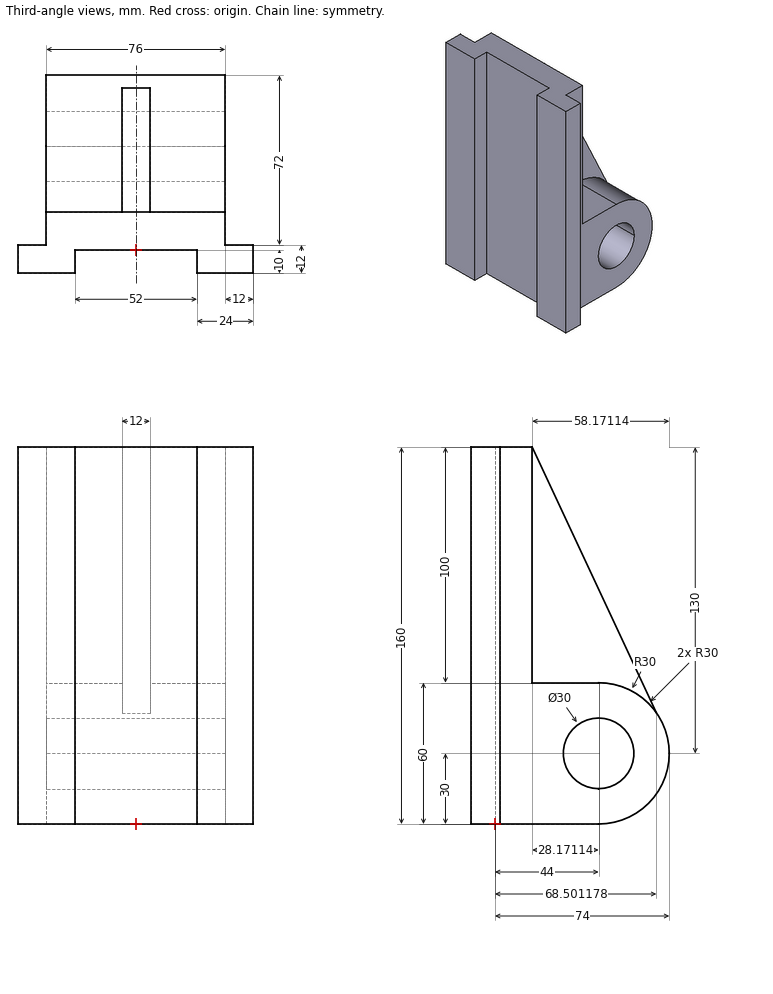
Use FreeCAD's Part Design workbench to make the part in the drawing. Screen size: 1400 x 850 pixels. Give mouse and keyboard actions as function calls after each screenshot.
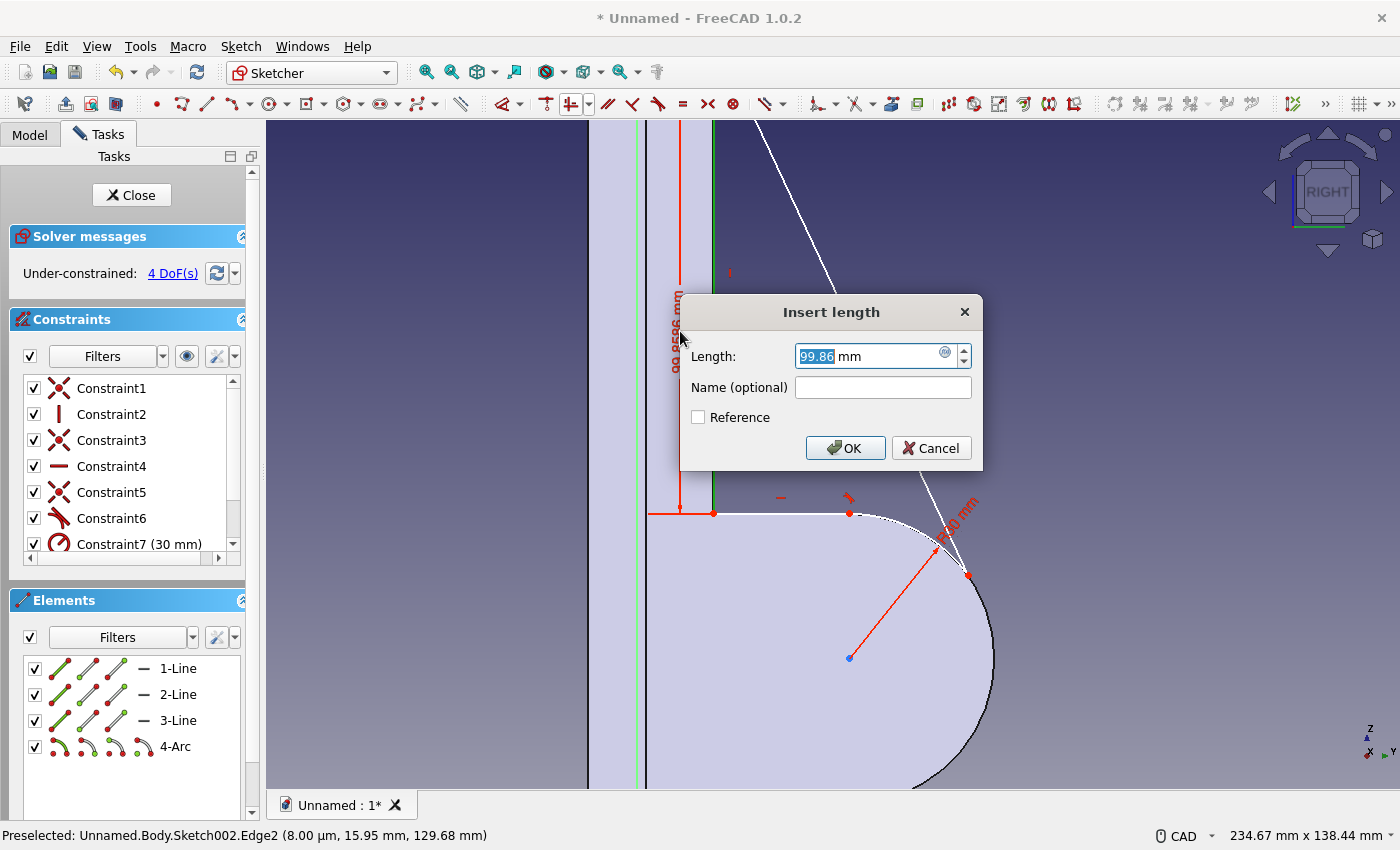
text(100)
key(Return)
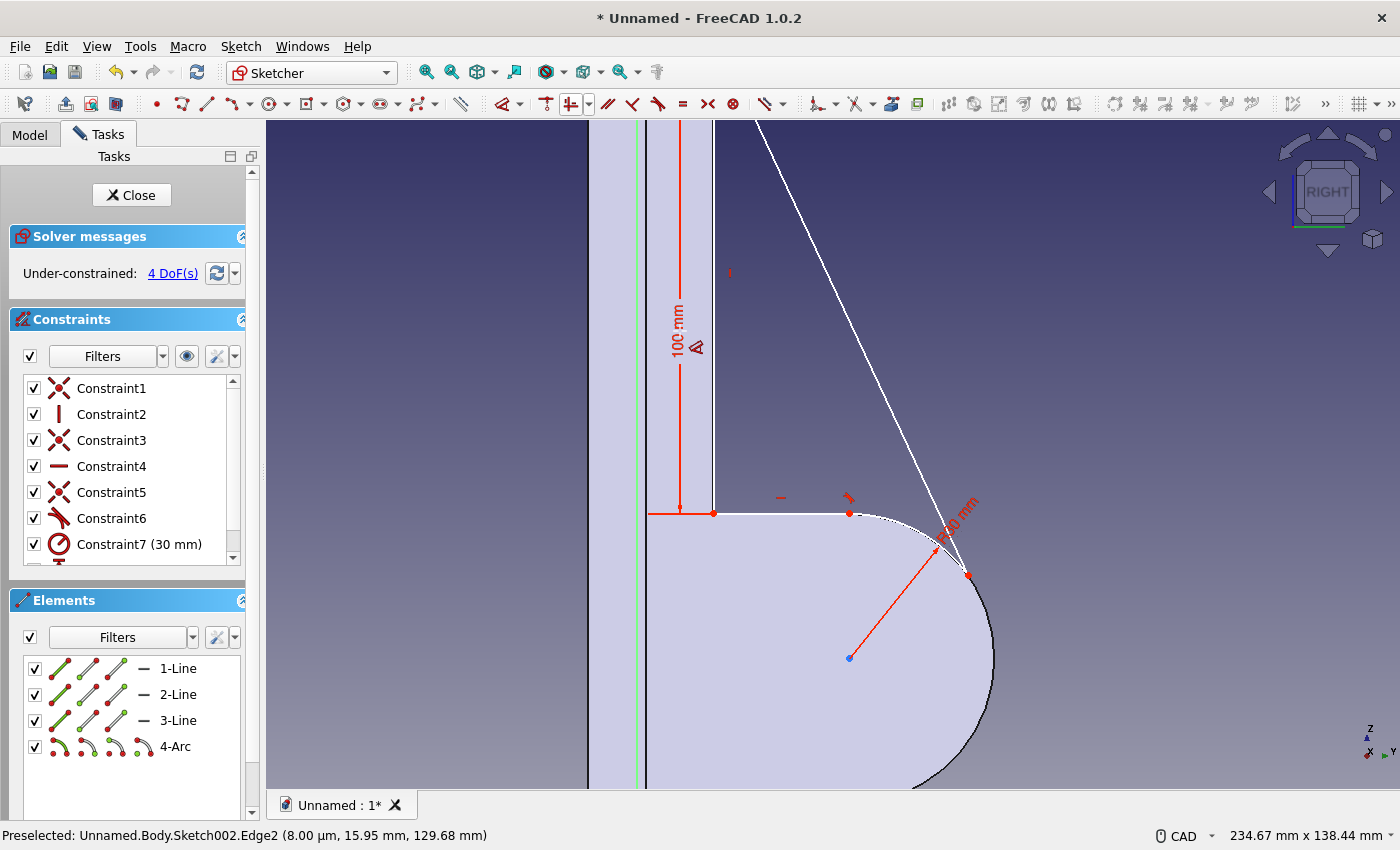
click(714, 514)
click(603, 637)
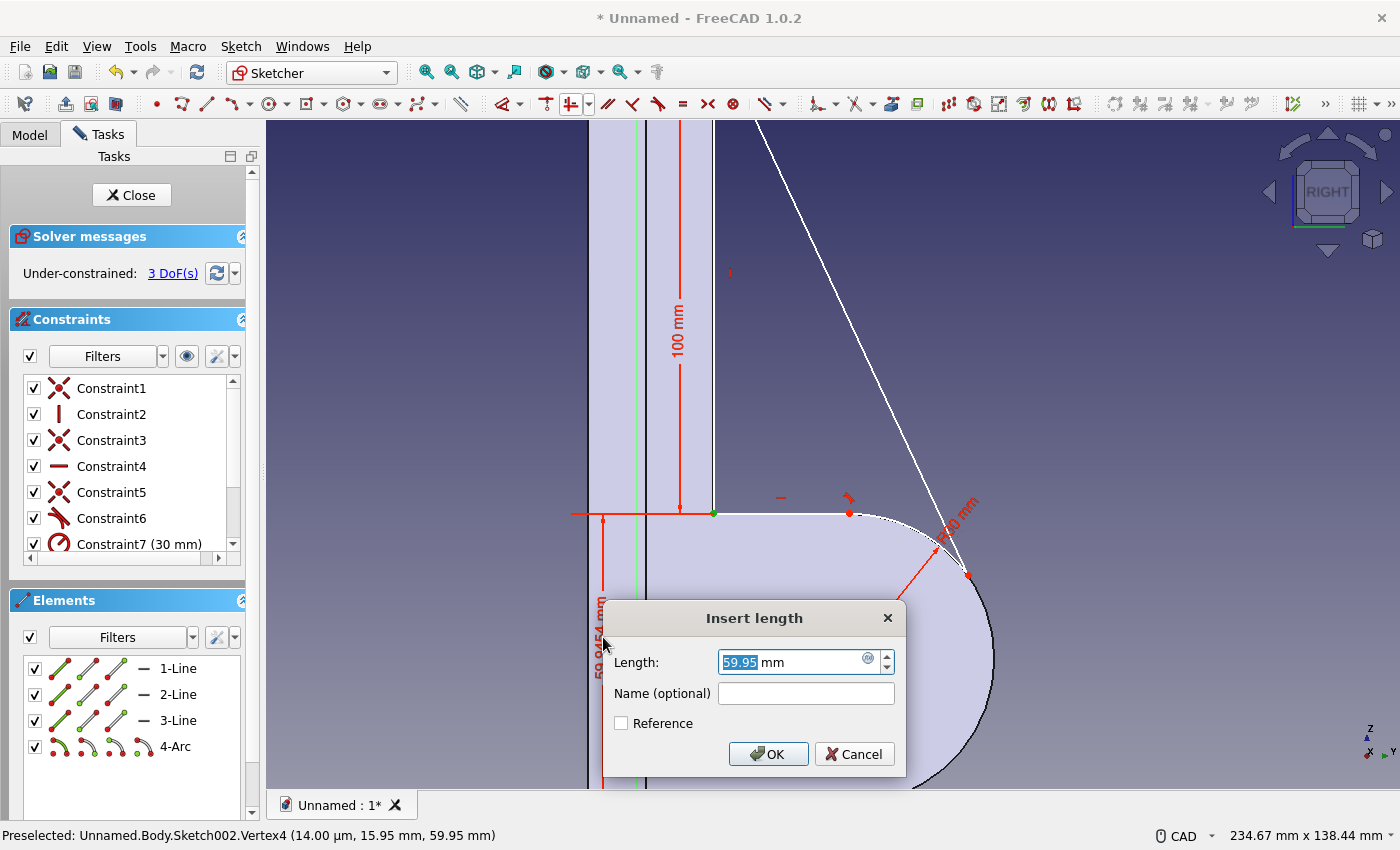
text(60)
key(Return)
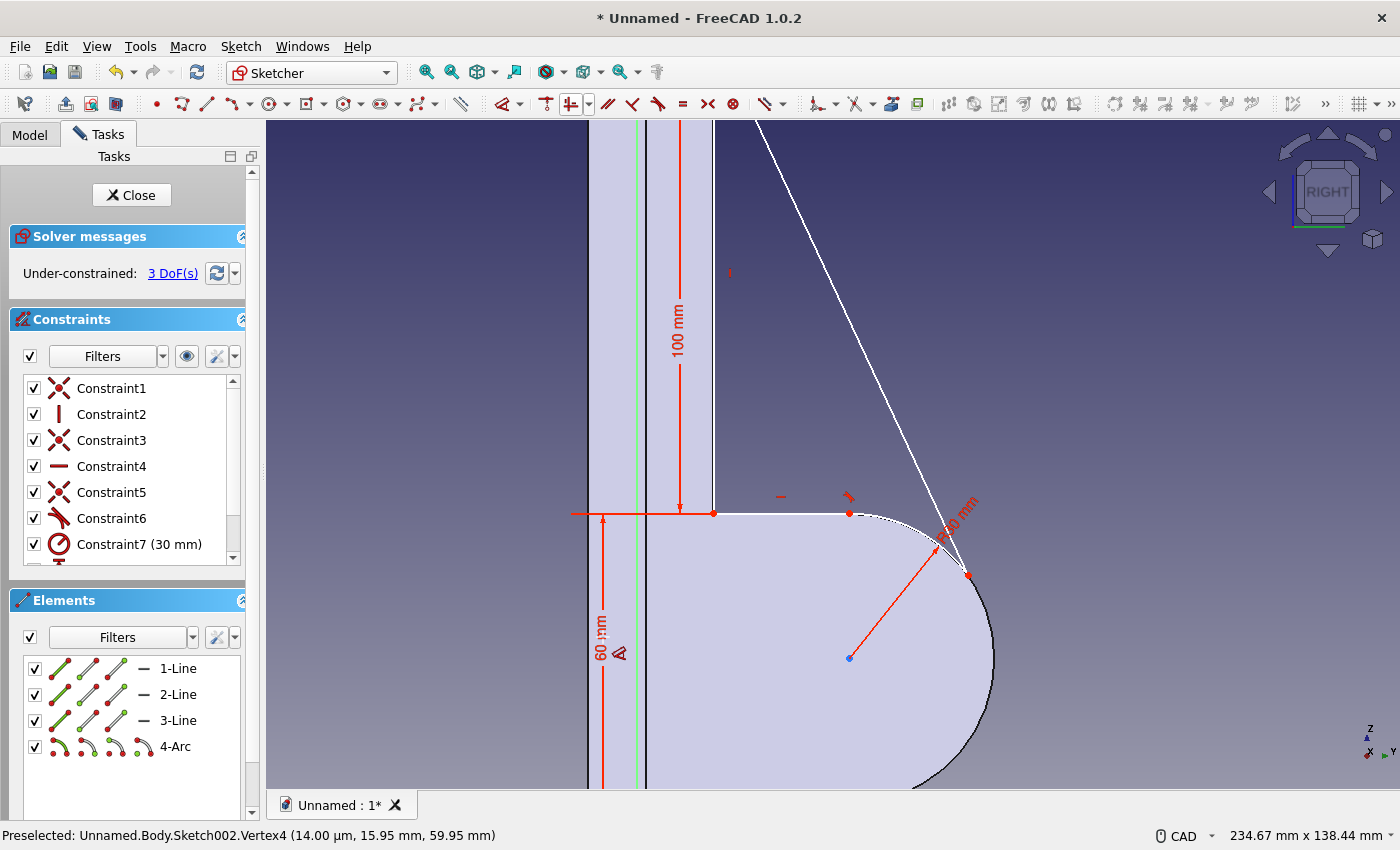
click(849, 514)
click(743, 480)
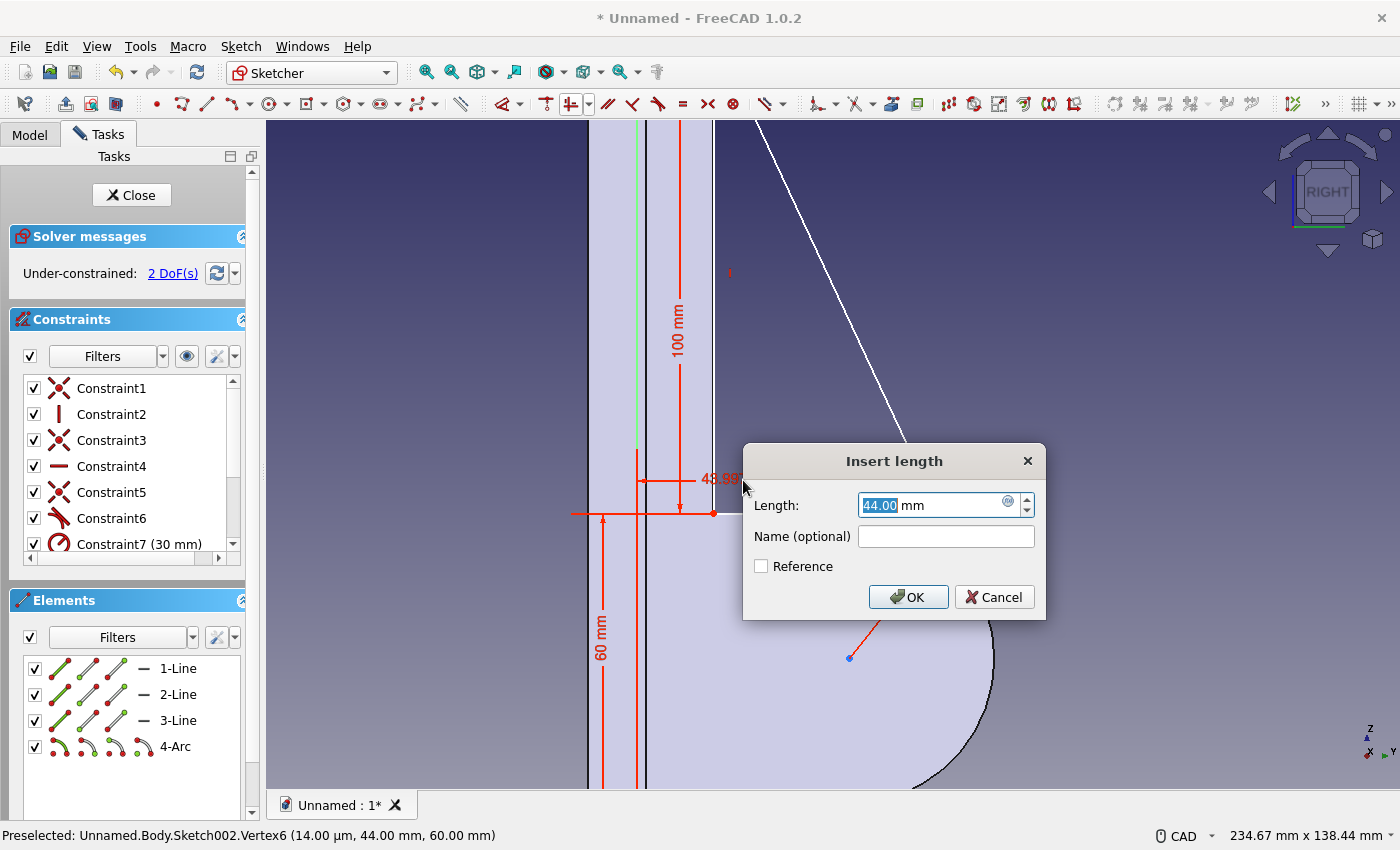
text(44)
key(Return)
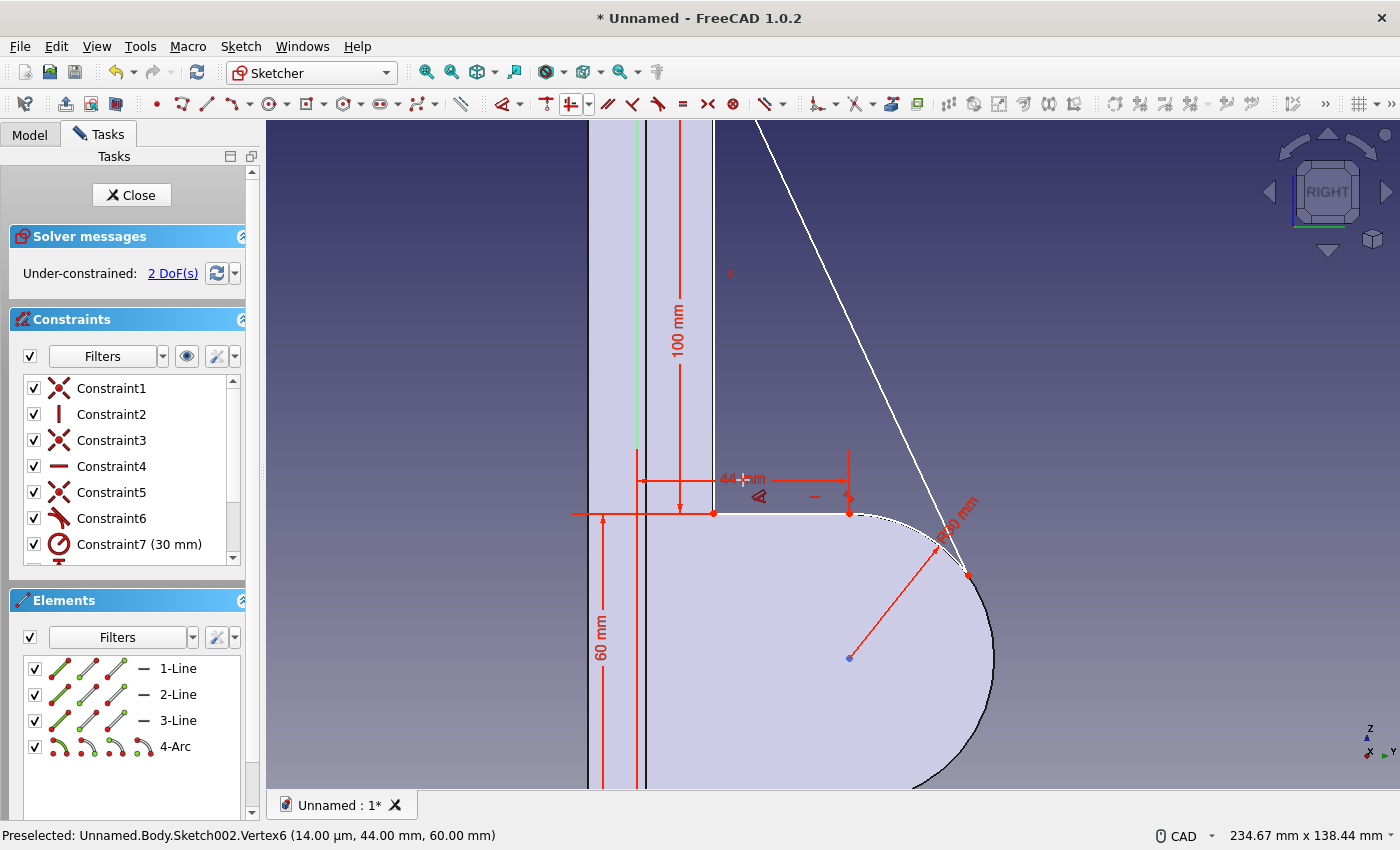
click(754, 514)
click(782, 548)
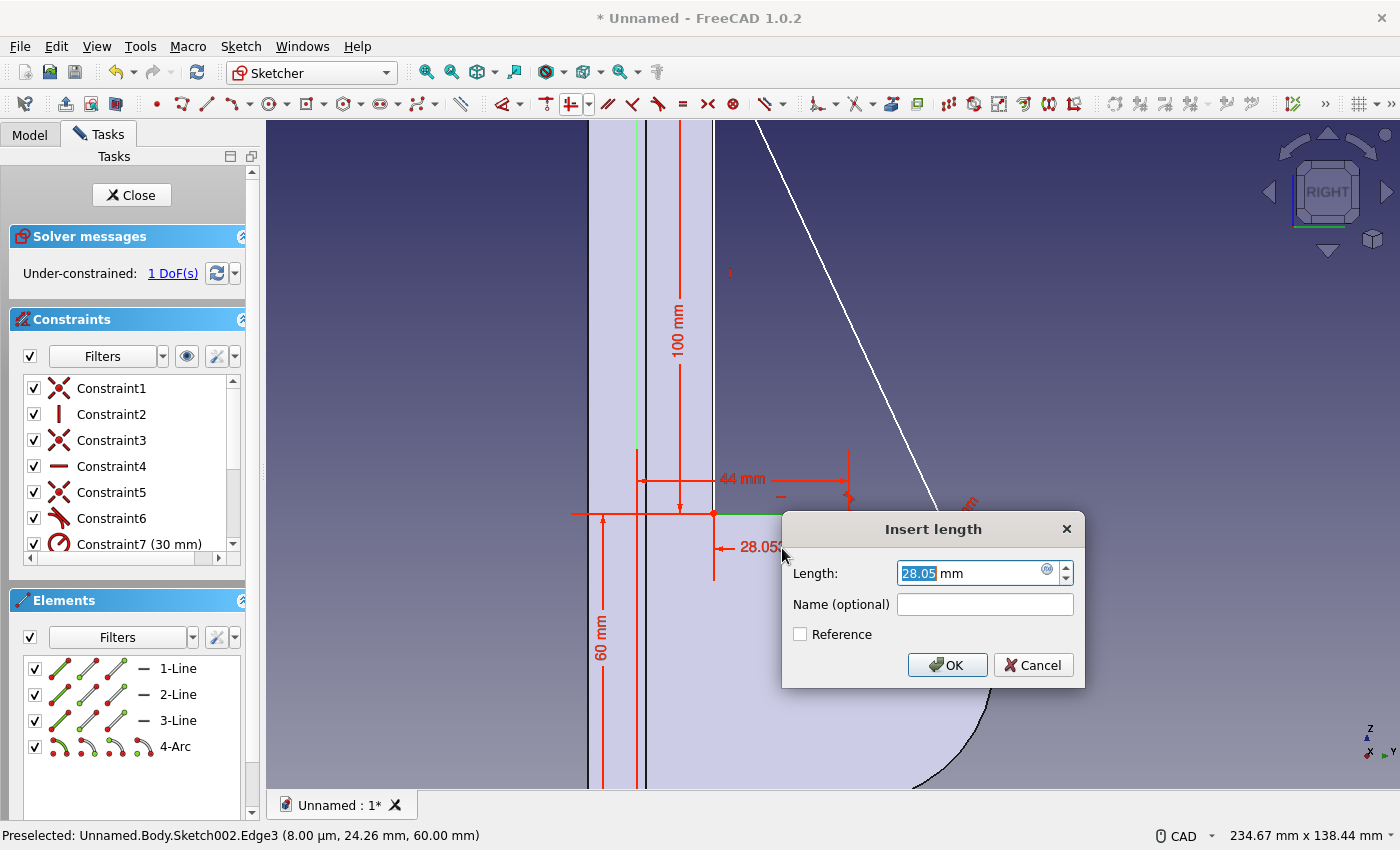
text(28.17114)
key(Return)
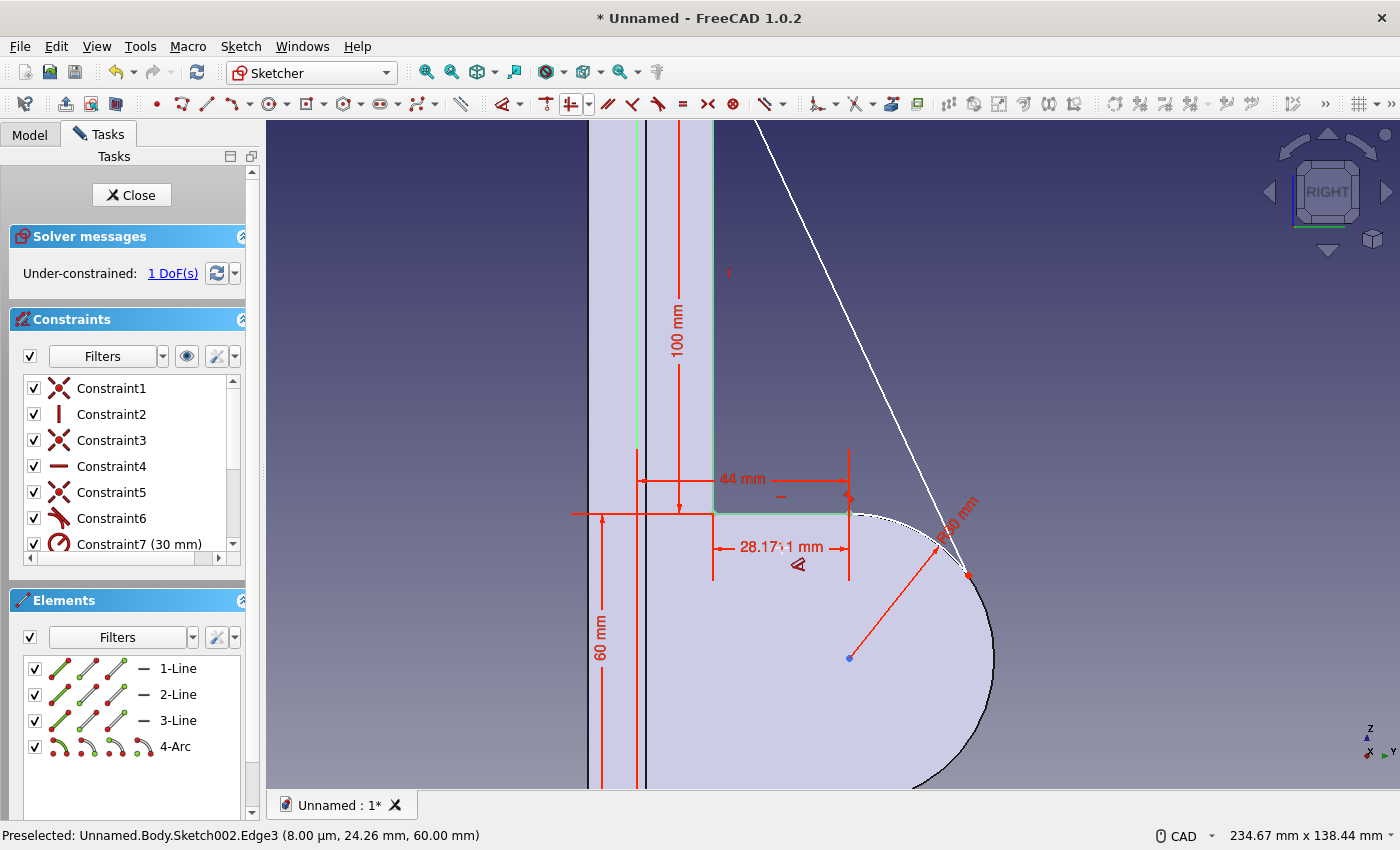
click(968, 576)
click(879, 542)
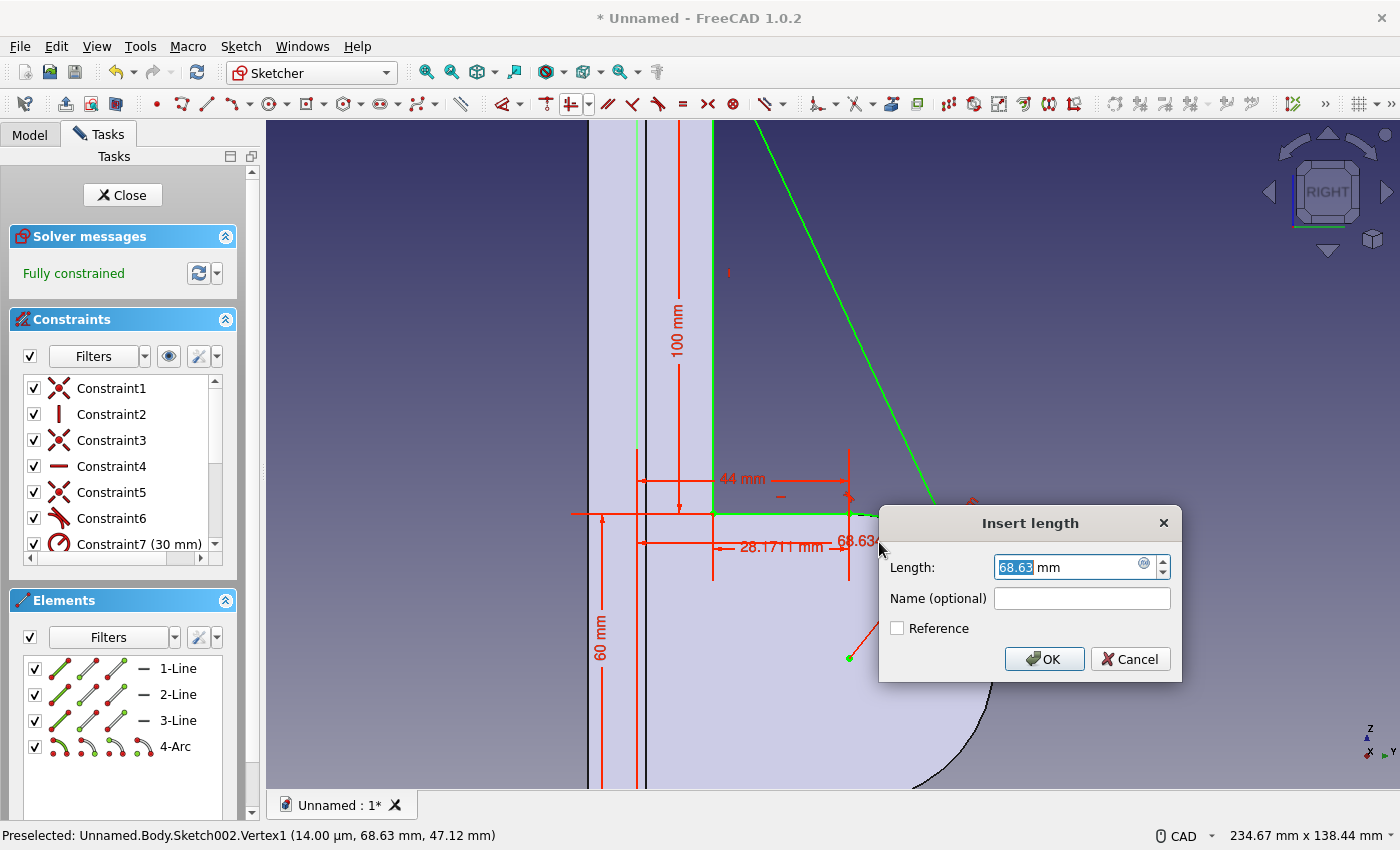
text(68.501178)
key(Return)
key(Escape)